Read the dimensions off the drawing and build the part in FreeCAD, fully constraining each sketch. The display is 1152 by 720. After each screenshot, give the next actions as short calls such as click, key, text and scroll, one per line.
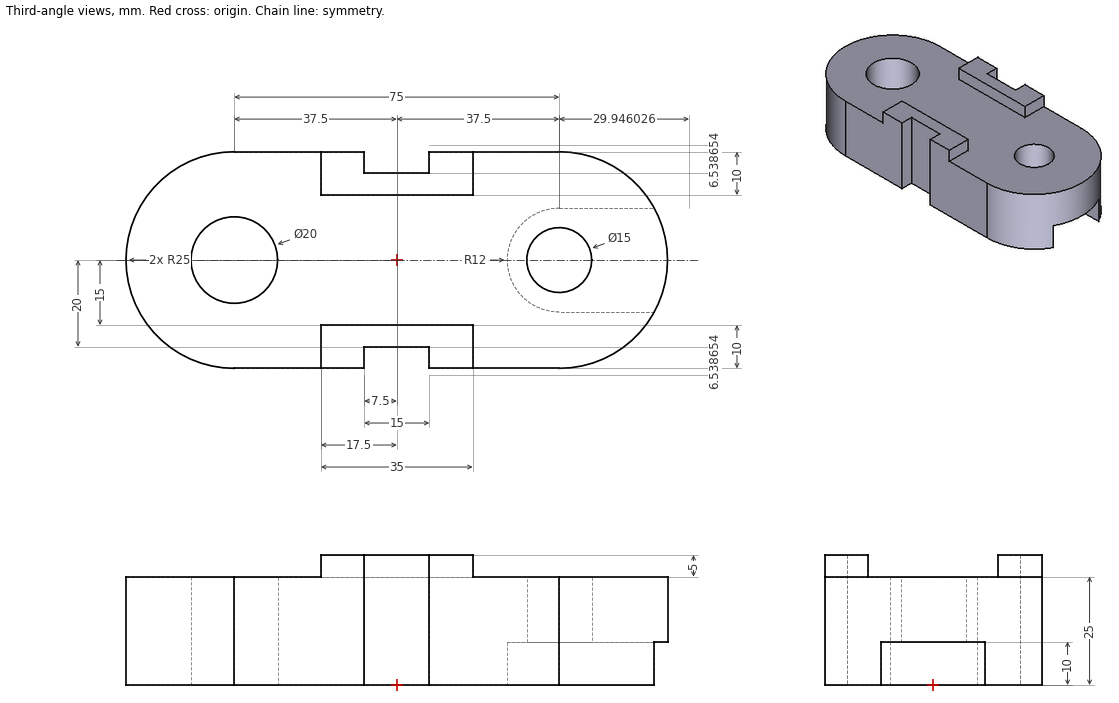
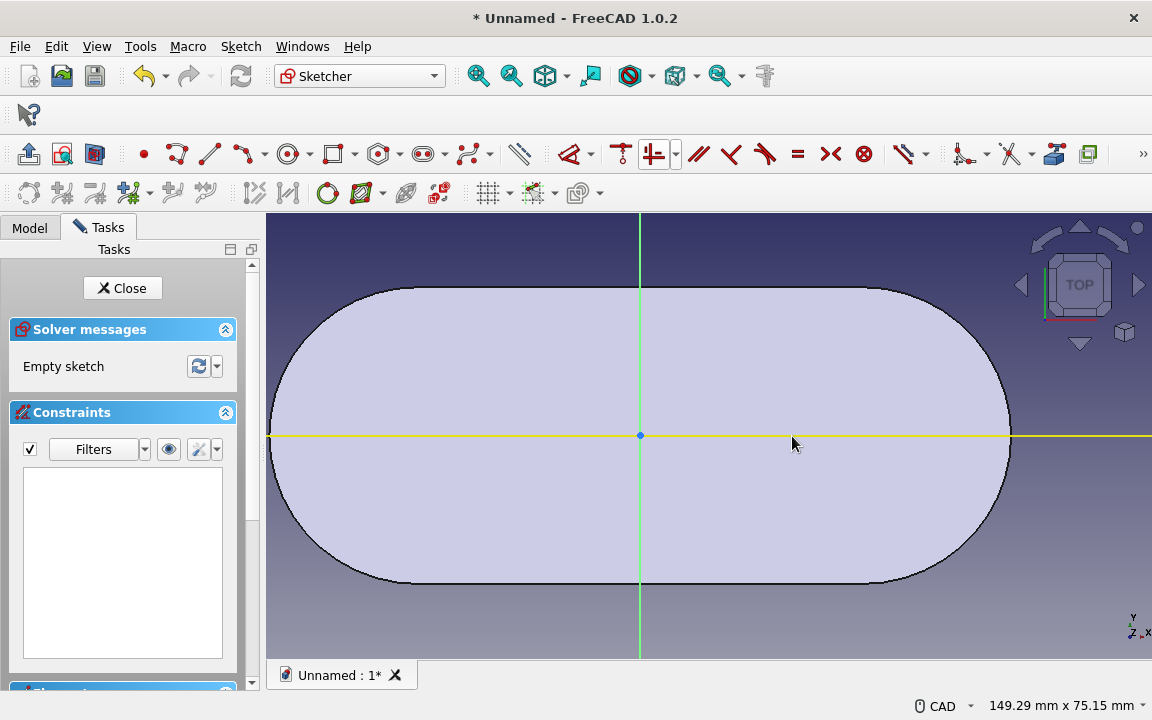
click(332, 154)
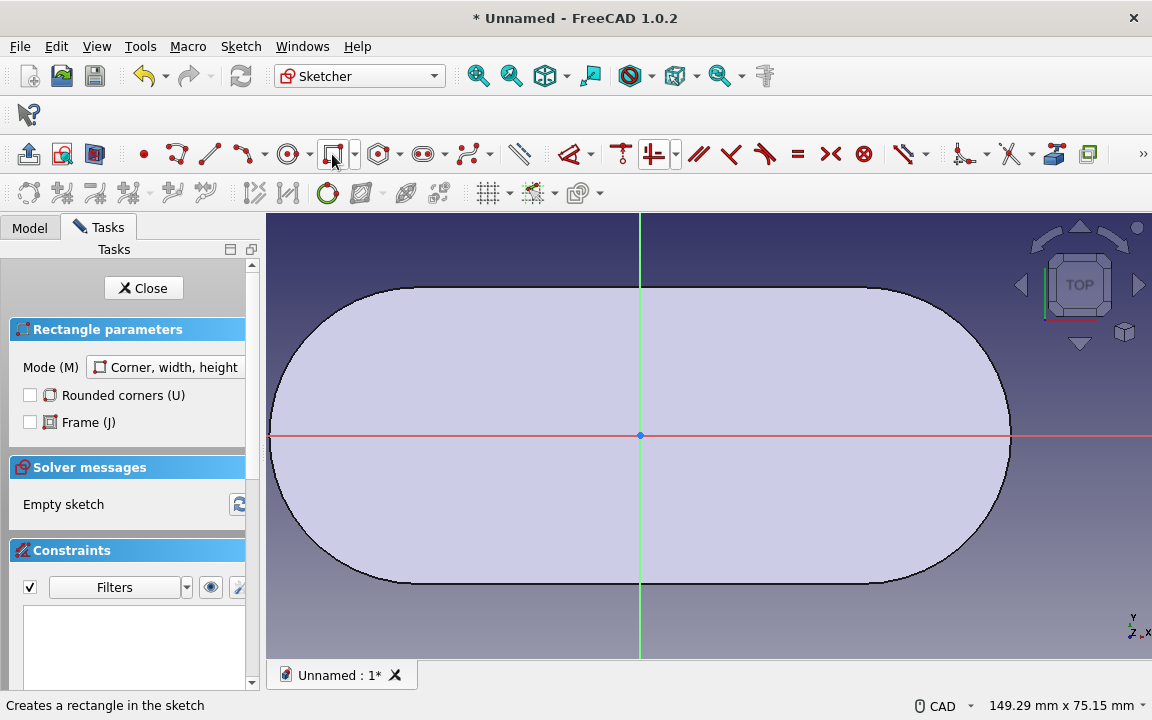
click(536, 525)
move(744, 584)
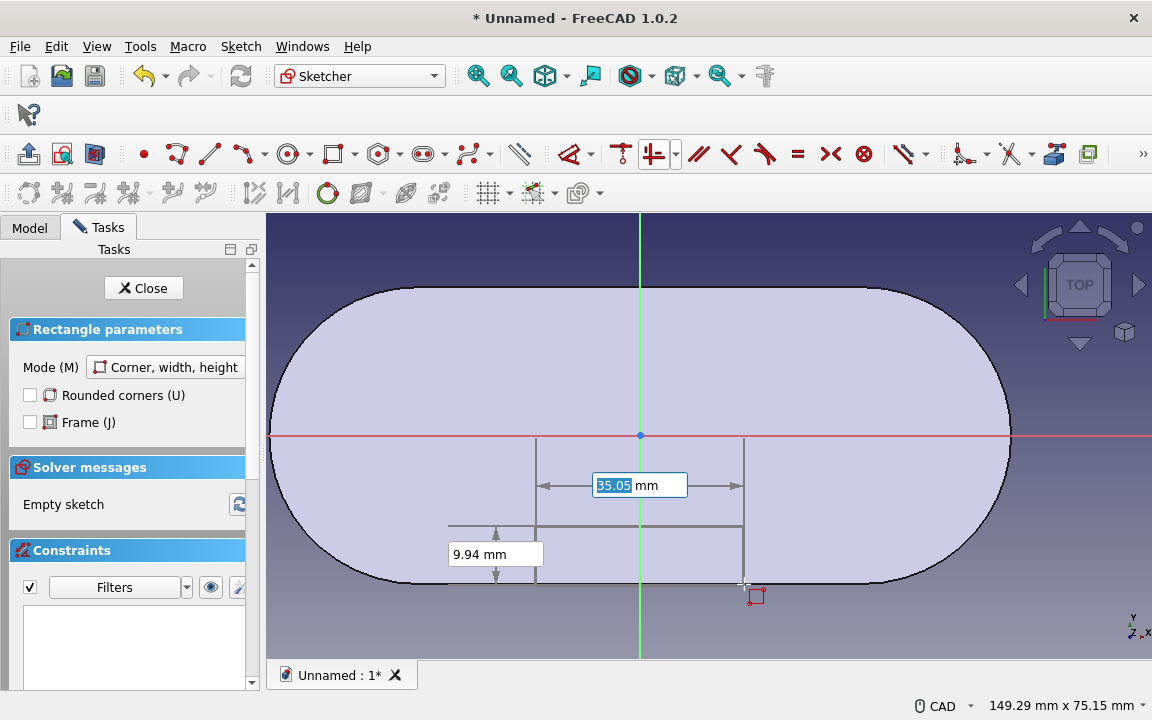
text(35)
key(Tab)
text(10)
key(Return)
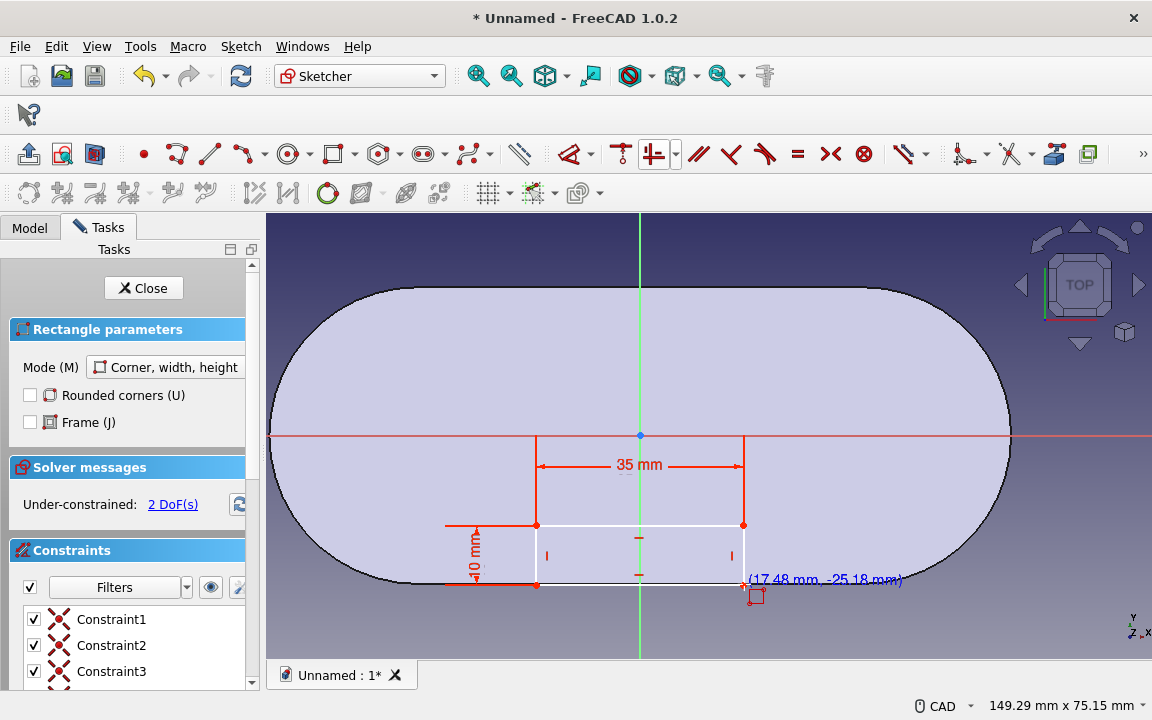
click(536, 287)
move(744, 347)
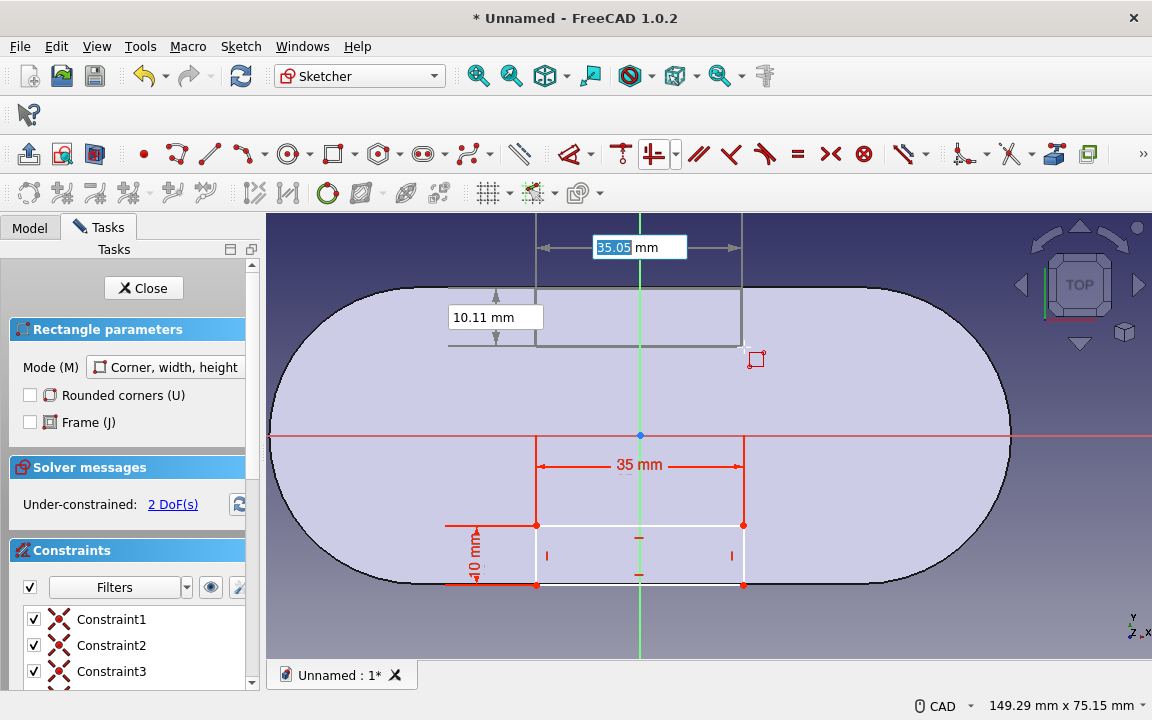
text(35)
key(Tab)
text(10)
key(Return)
key(Escape)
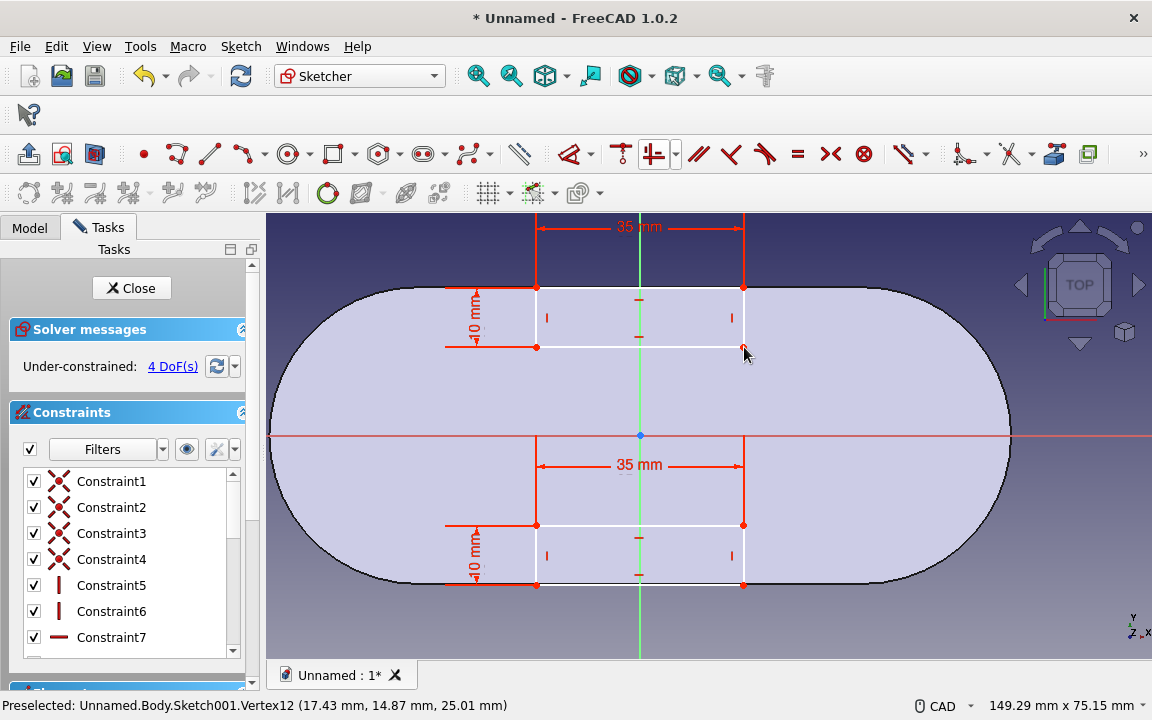
click(536, 585)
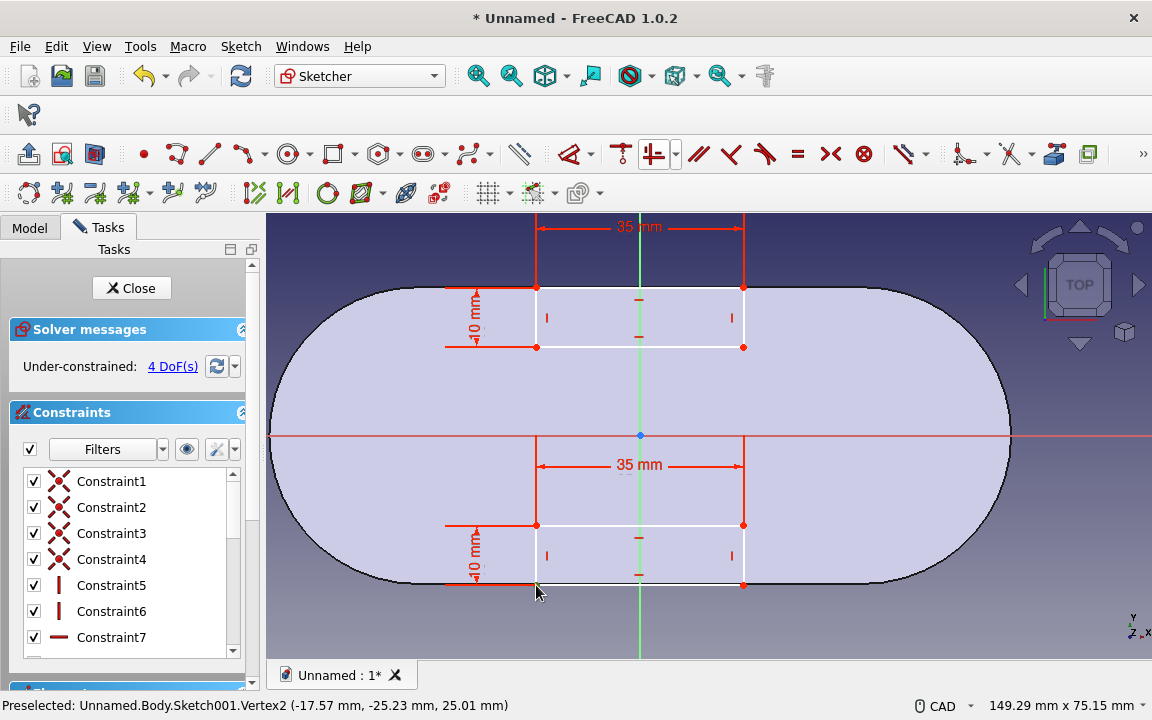
click(536, 288)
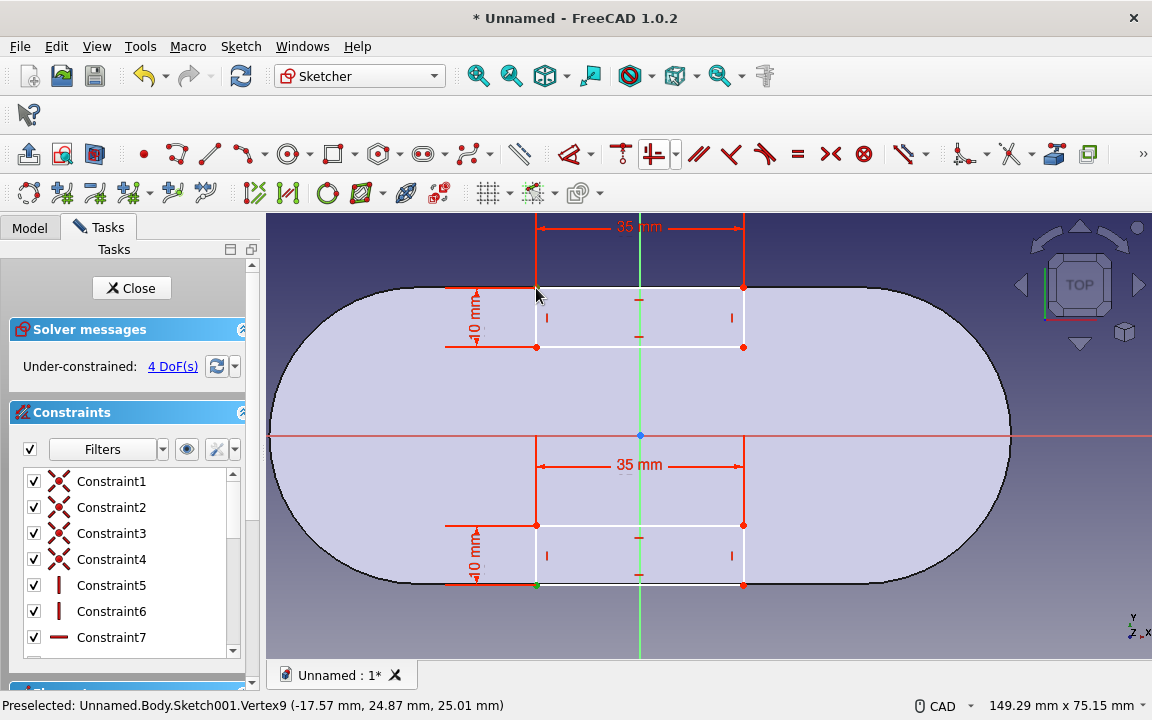
click(344, 436)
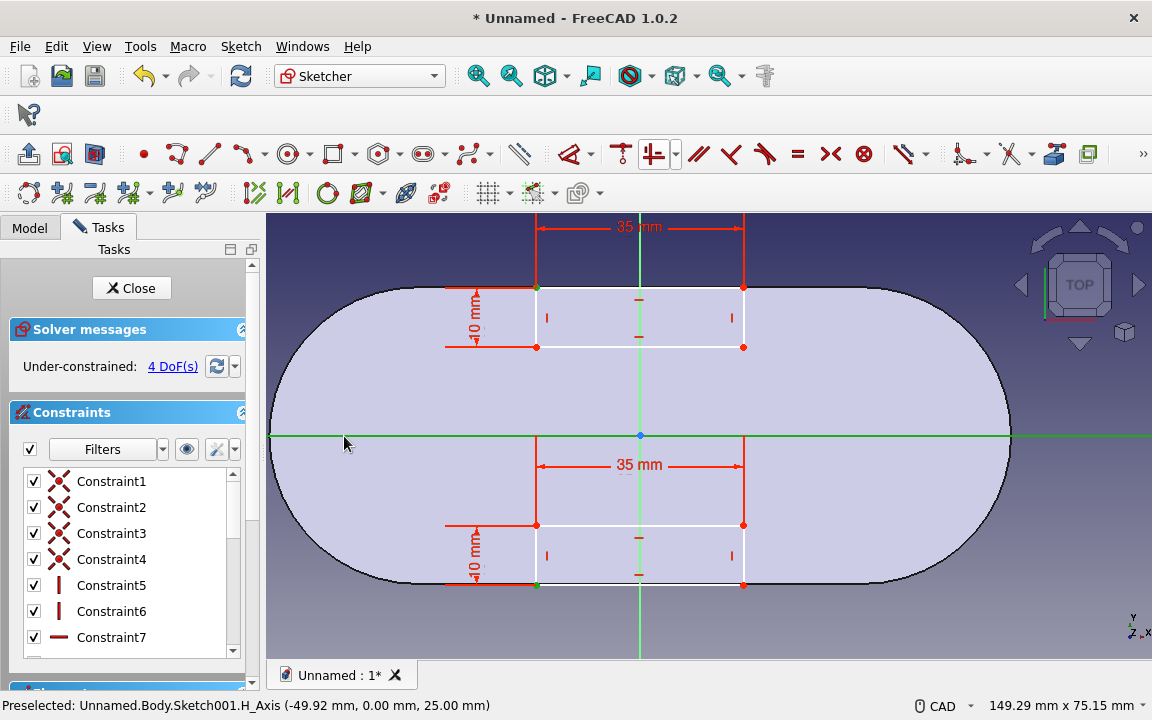
click(831, 154)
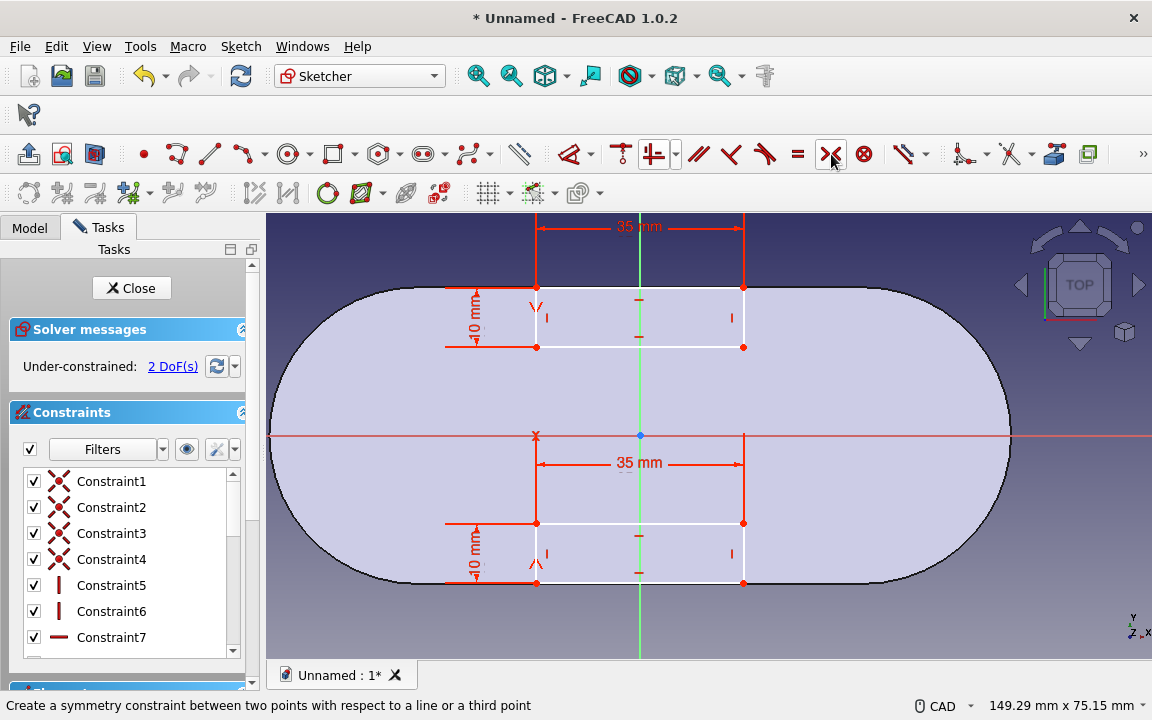
click(568, 154)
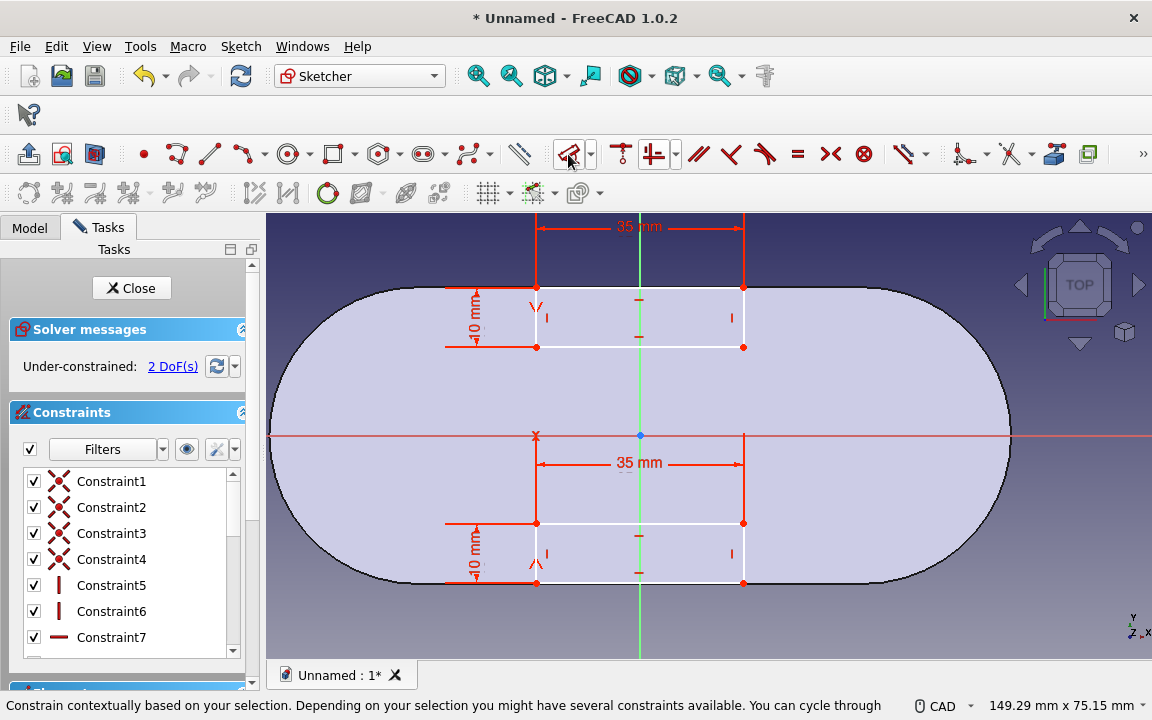
click(536, 524)
click(502, 480)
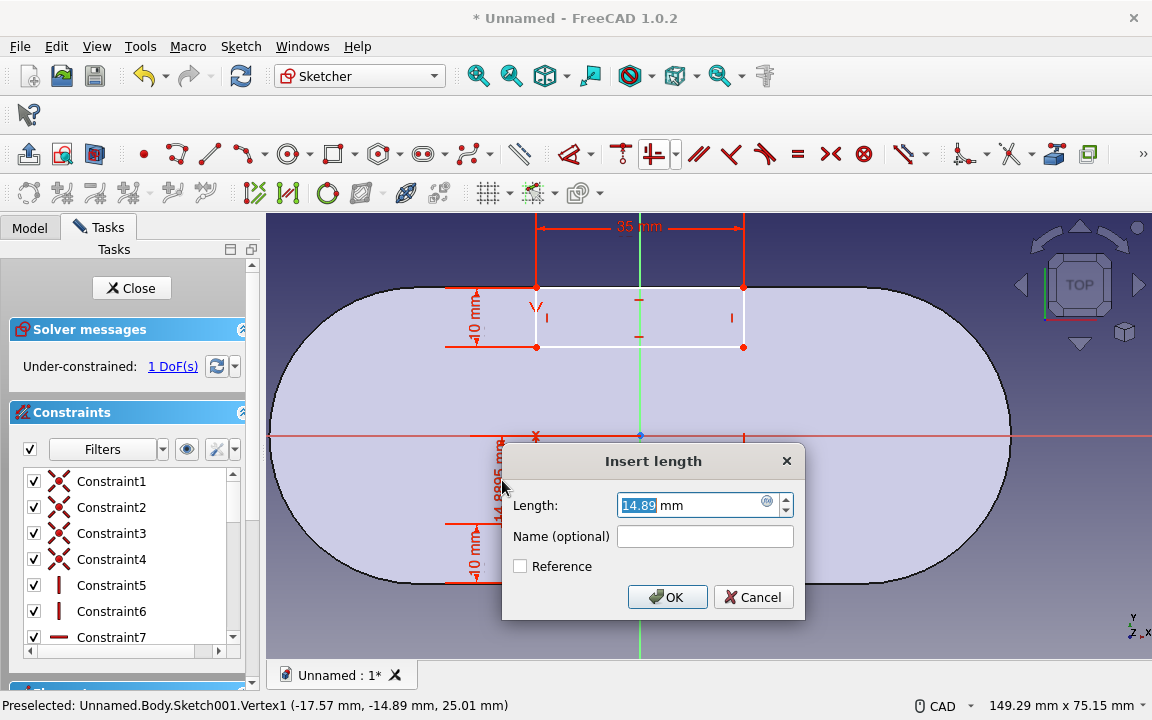
text(15)
key(Return)